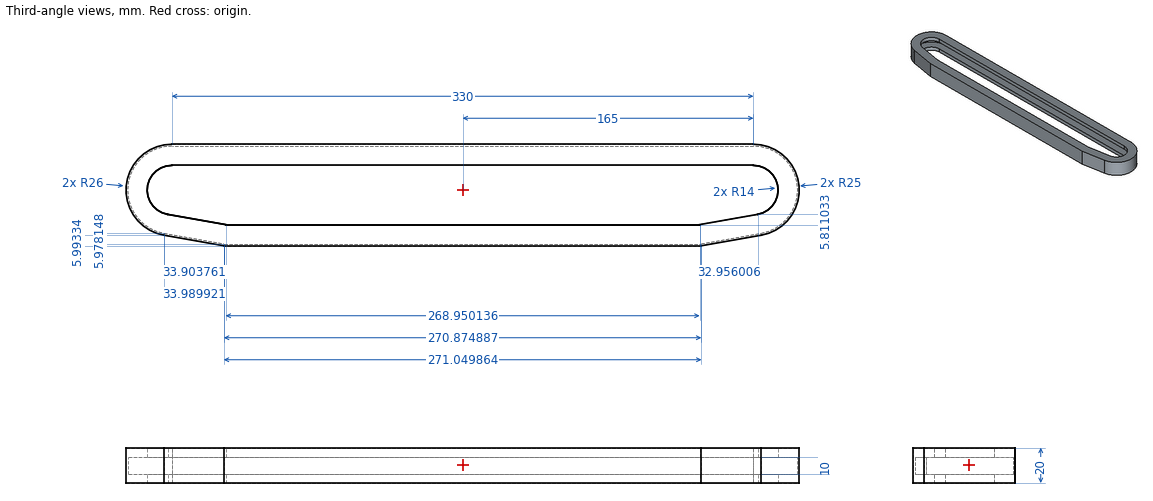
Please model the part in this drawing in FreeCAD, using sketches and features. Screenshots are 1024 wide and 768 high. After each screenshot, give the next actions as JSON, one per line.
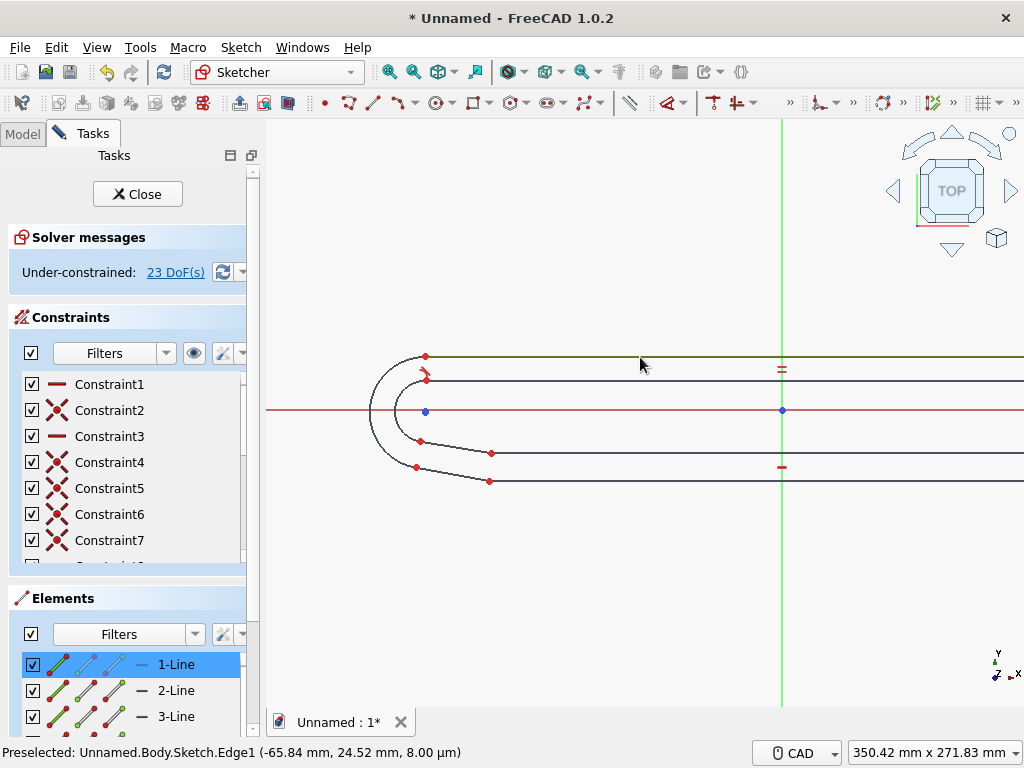
{"action": "scroll", "coordinate": [408, 411], "scroll_direction": "down", "scroll_amount": 4}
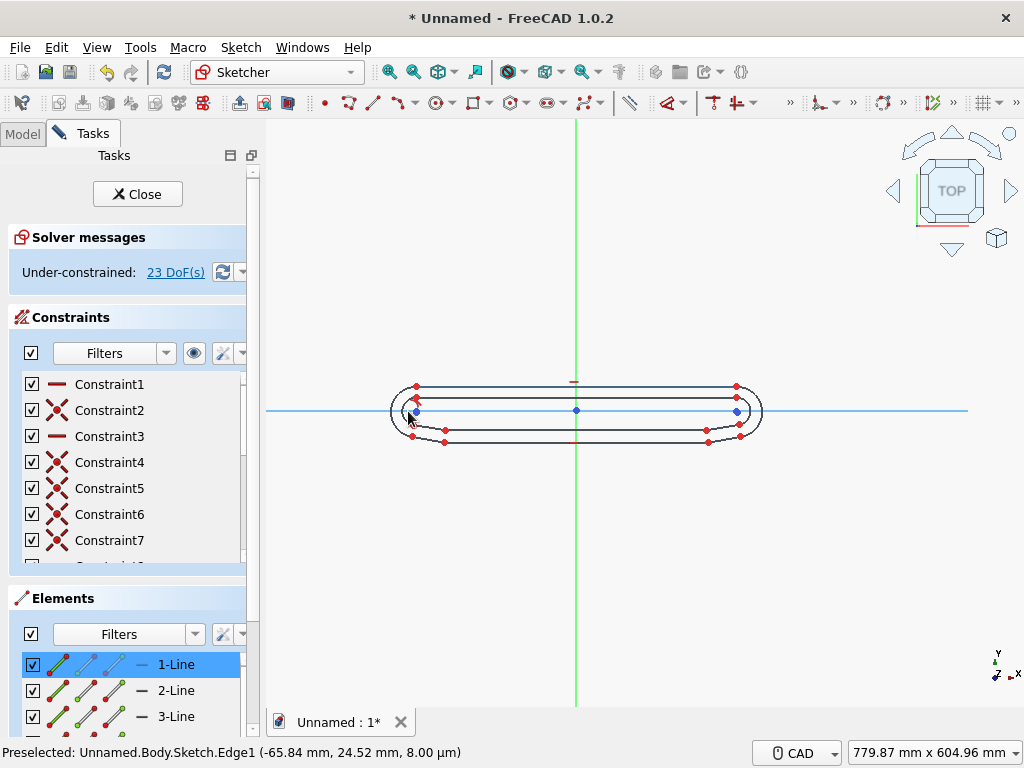
{"action": "left_click", "coordinate": [759, 424]}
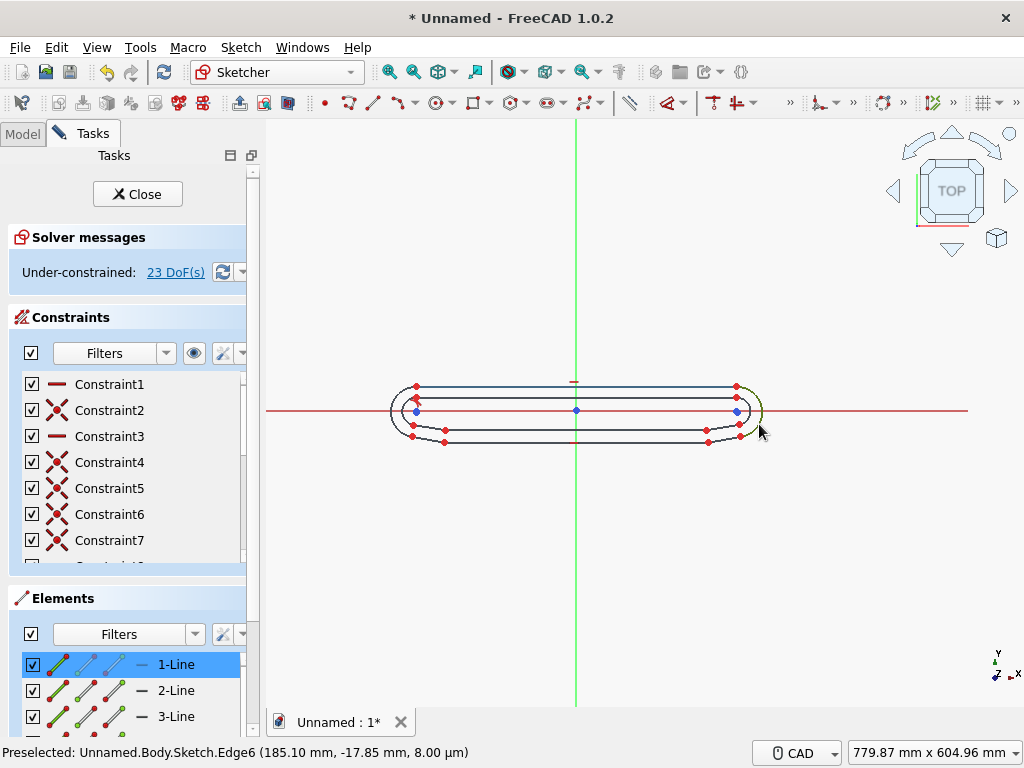
{"action": "key", "text": "t"}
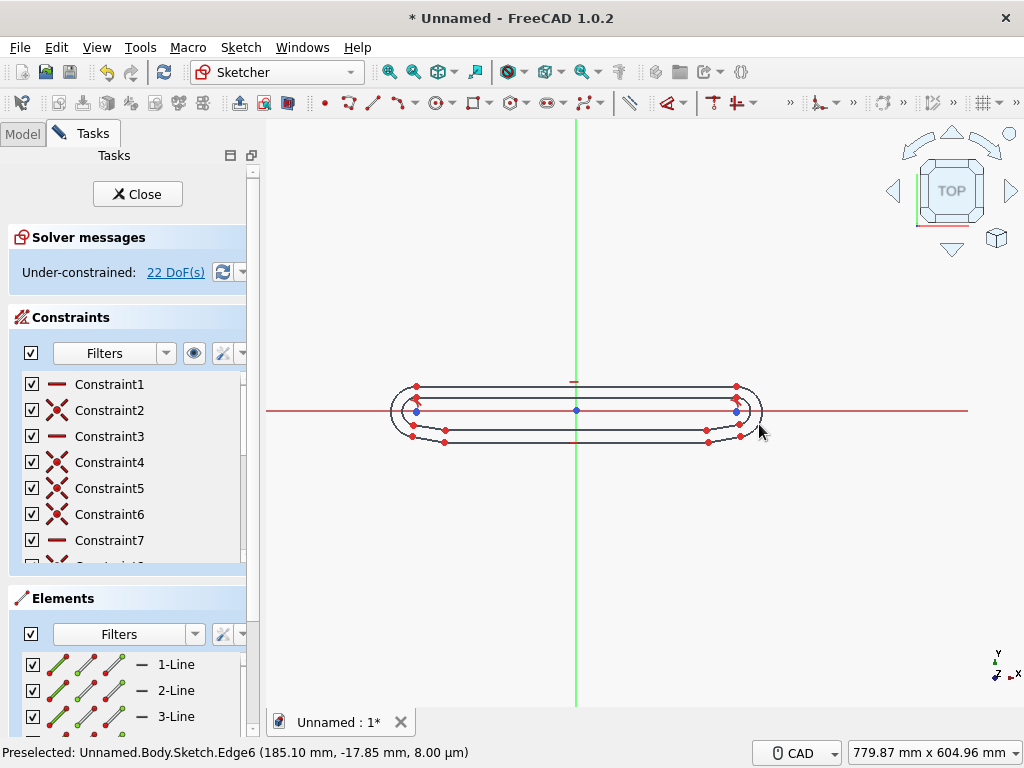
{"action": "scroll", "coordinate": [422, 439], "scroll_direction": "up", "scroll_amount": 2}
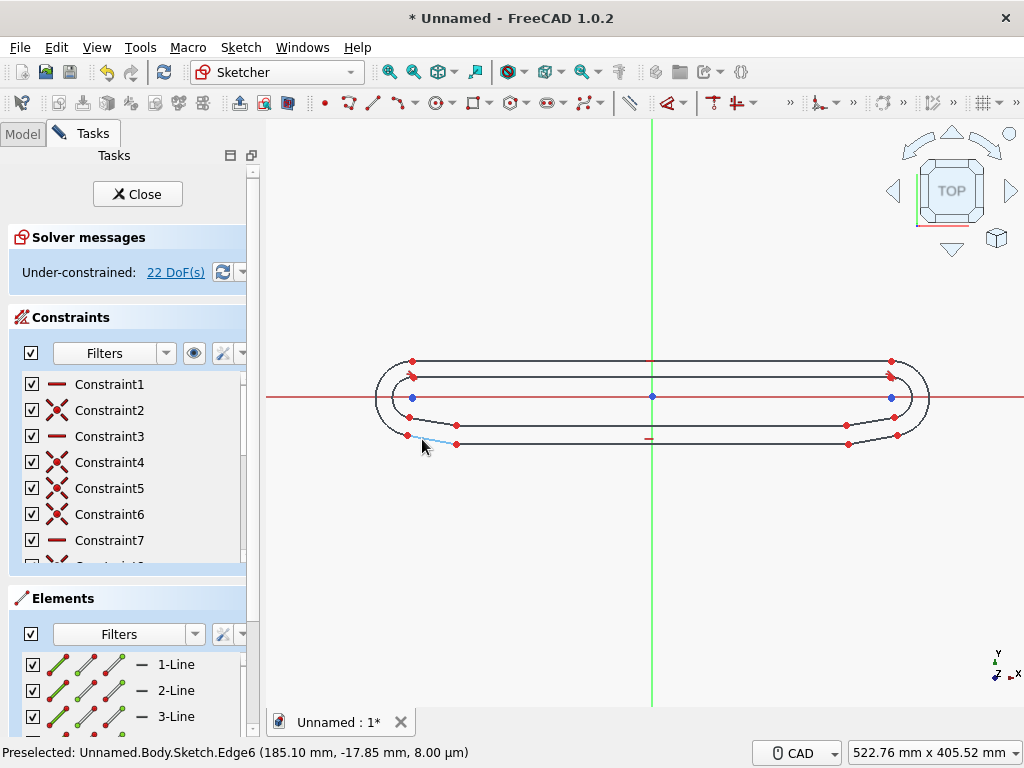
{"action": "left_click", "coordinate": [422, 438]}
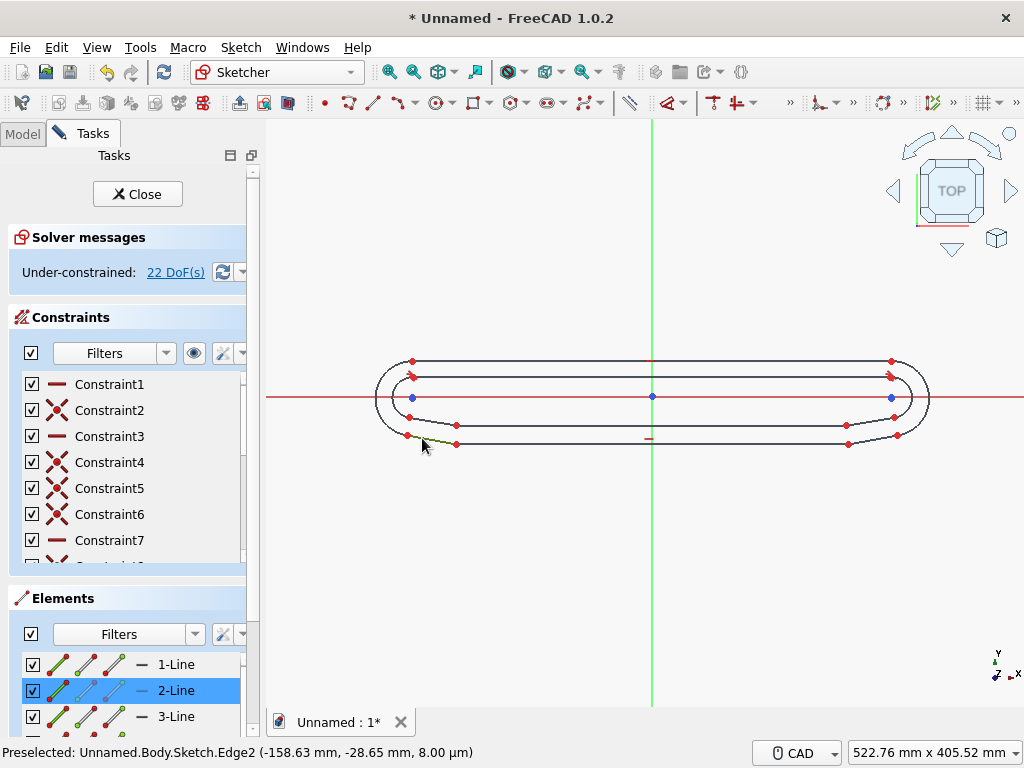
{"action": "left_click", "coordinate": [384, 375]}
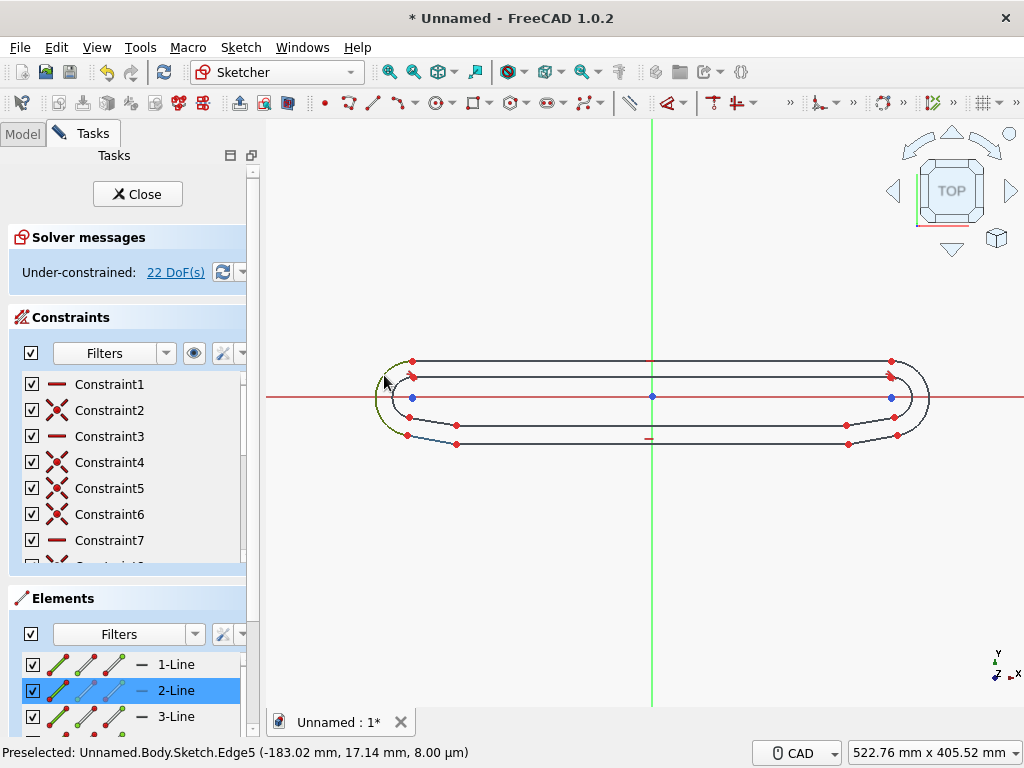
{"action": "key", "text": "t"}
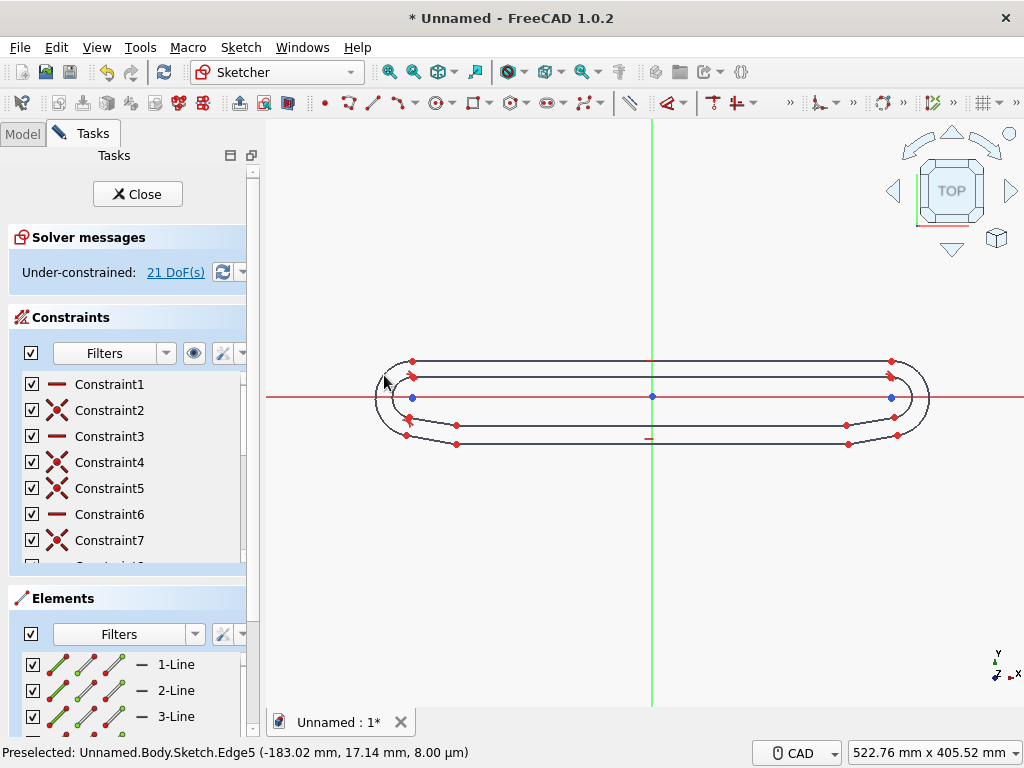
{"action": "scroll", "coordinate": [858, 443], "scroll_direction": "up", "scroll_amount": 2}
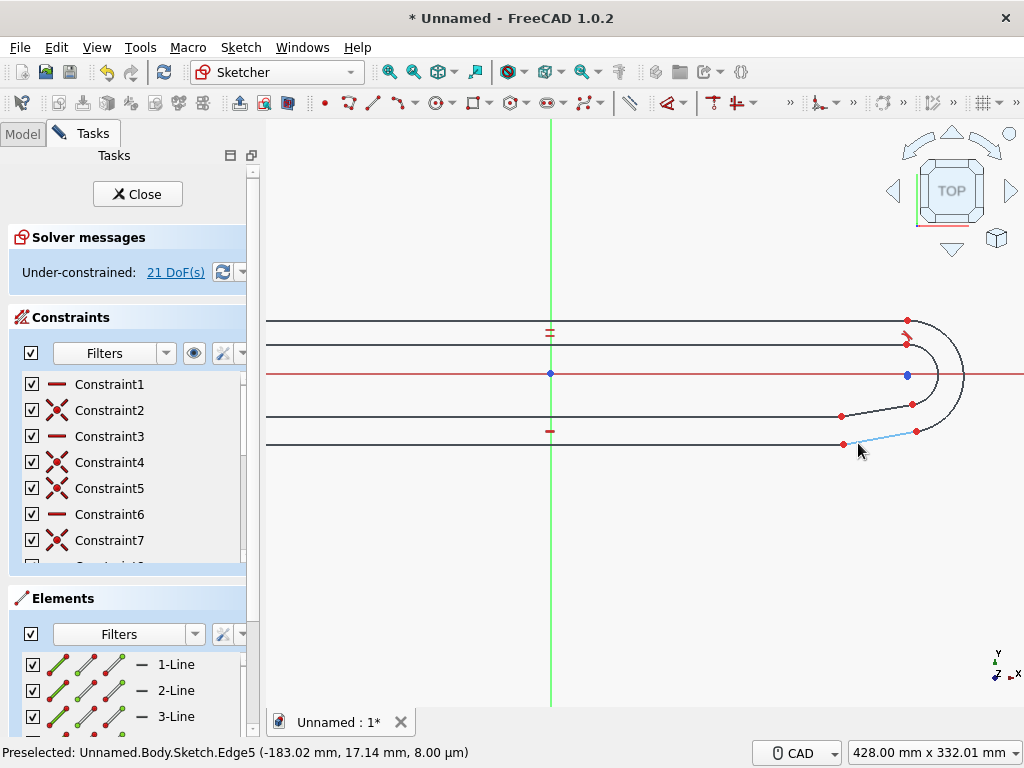
{"action": "left_click", "coordinate": [858, 442]}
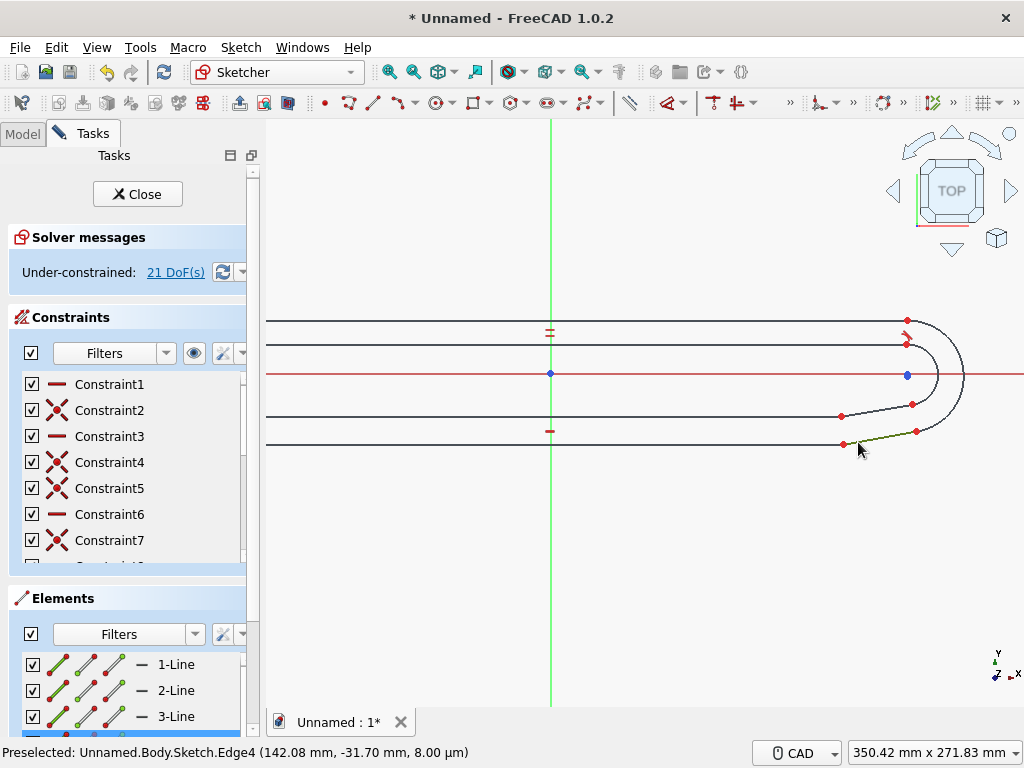
{"action": "scroll", "coordinate": [598, 440], "scroll_direction": "down", "scroll_amount": 4}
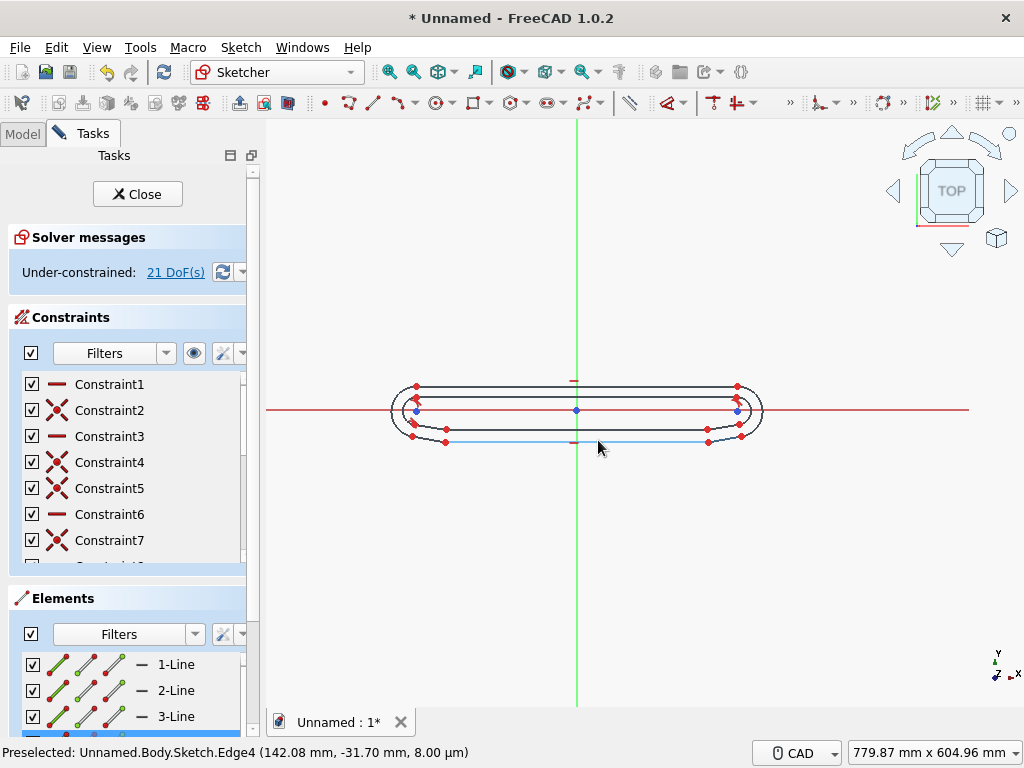
{"action": "left_click", "coordinate": [759, 424]}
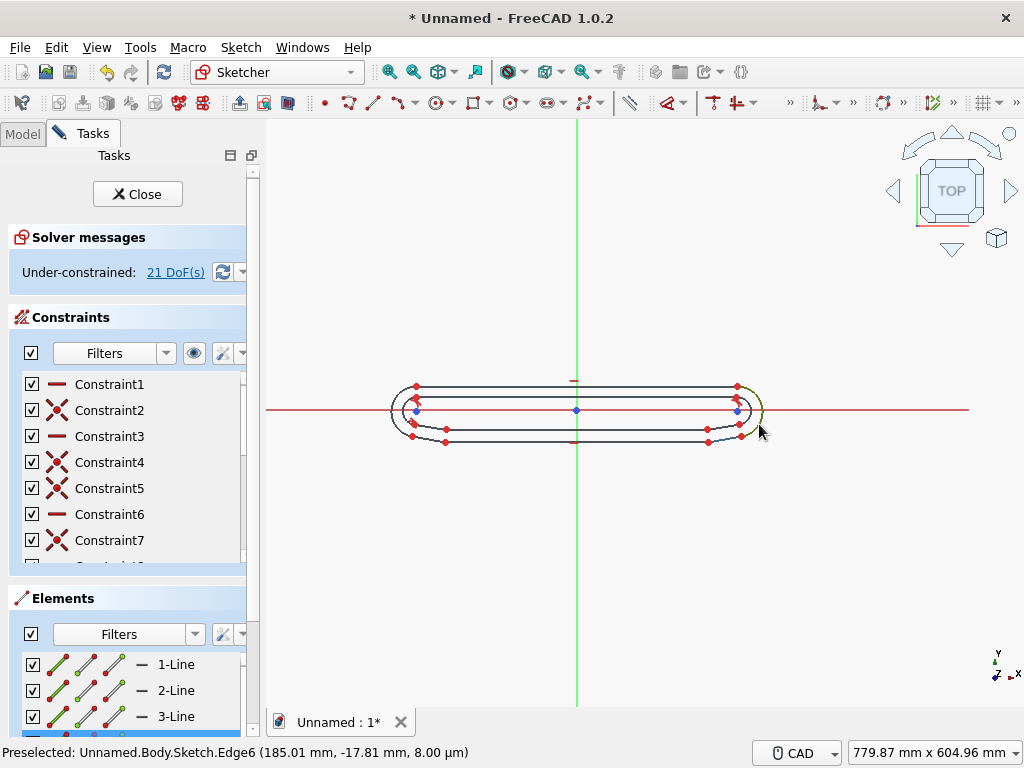
{"action": "key", "text": "t"}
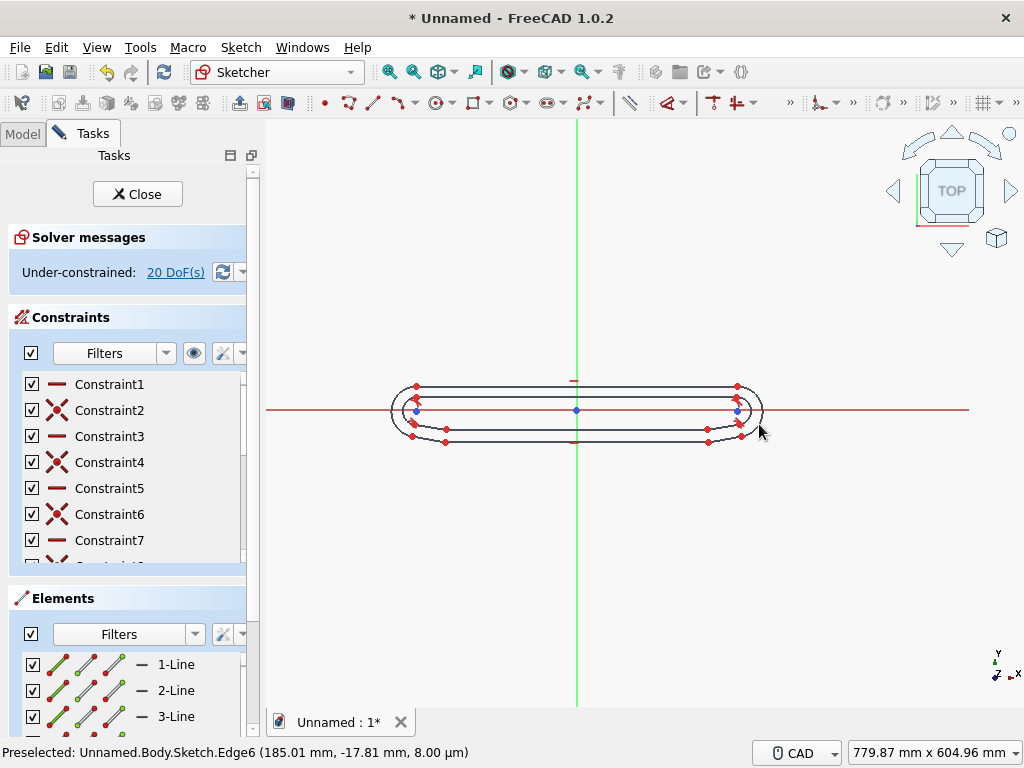
{"action": "scroll", "coordinate": [513, 397], "scroll_direction": "up", "scroll_amount": 2}